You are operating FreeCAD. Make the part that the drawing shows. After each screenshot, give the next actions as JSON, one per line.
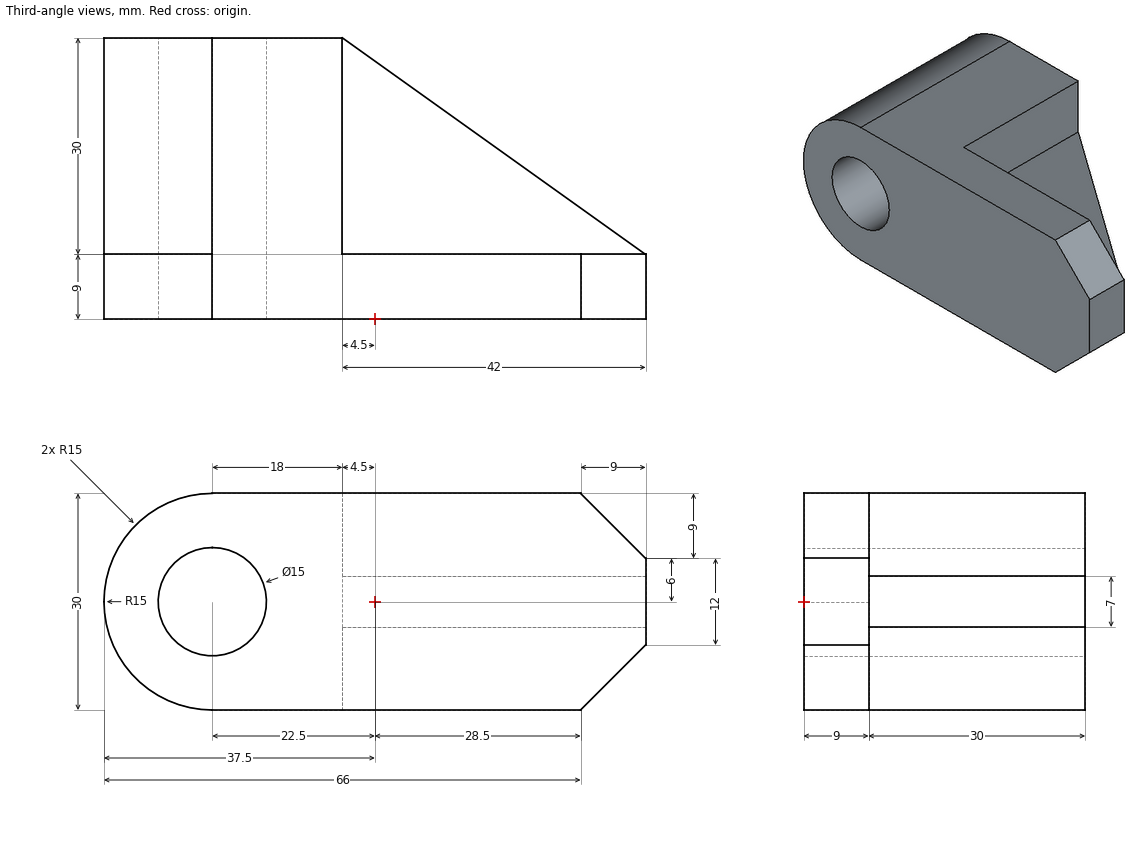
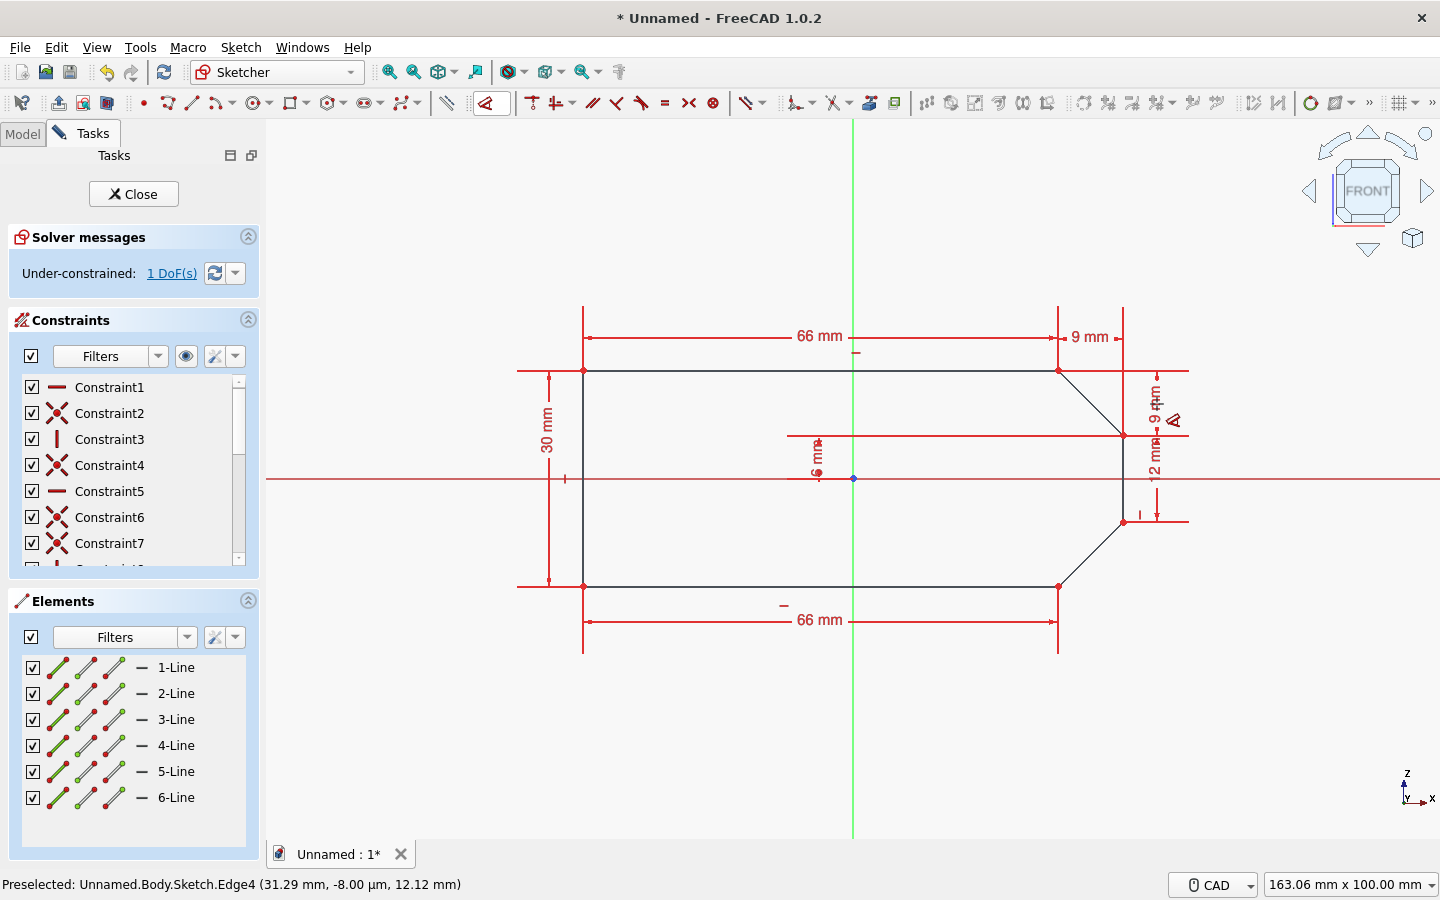
{"action": "left_click", "coordinate": [1058, 587]}
{"action": "left_click", "coordinate": [956, 621]}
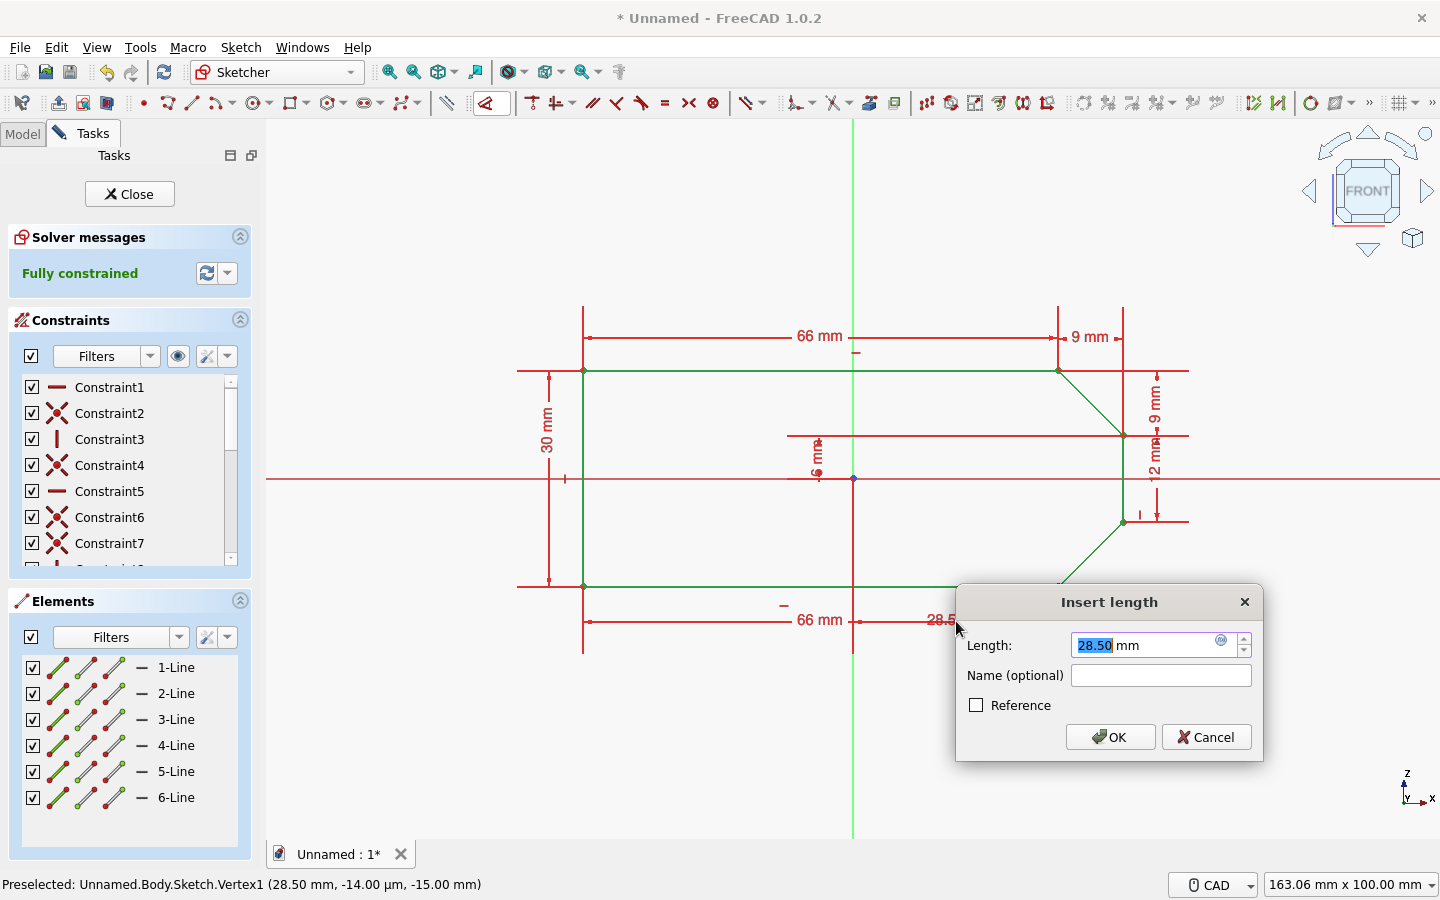
{"action": "type", "text": "28.5"}
{"action": "key", "text": "Return"}
{"action": "key", "text": "Escape"}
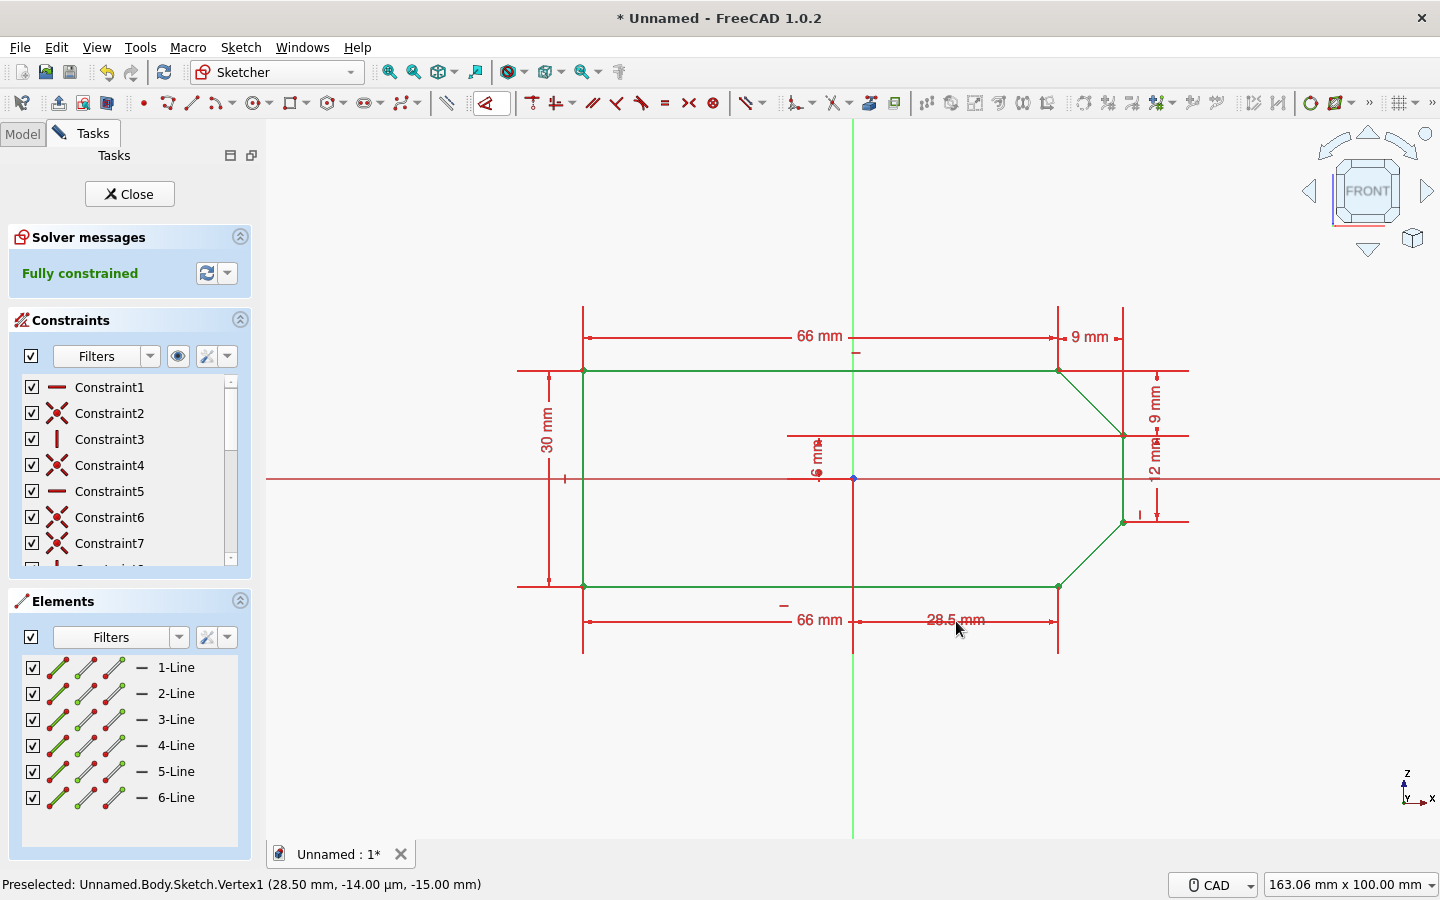
{"action": "left_click", "coordinate": [130, 194]}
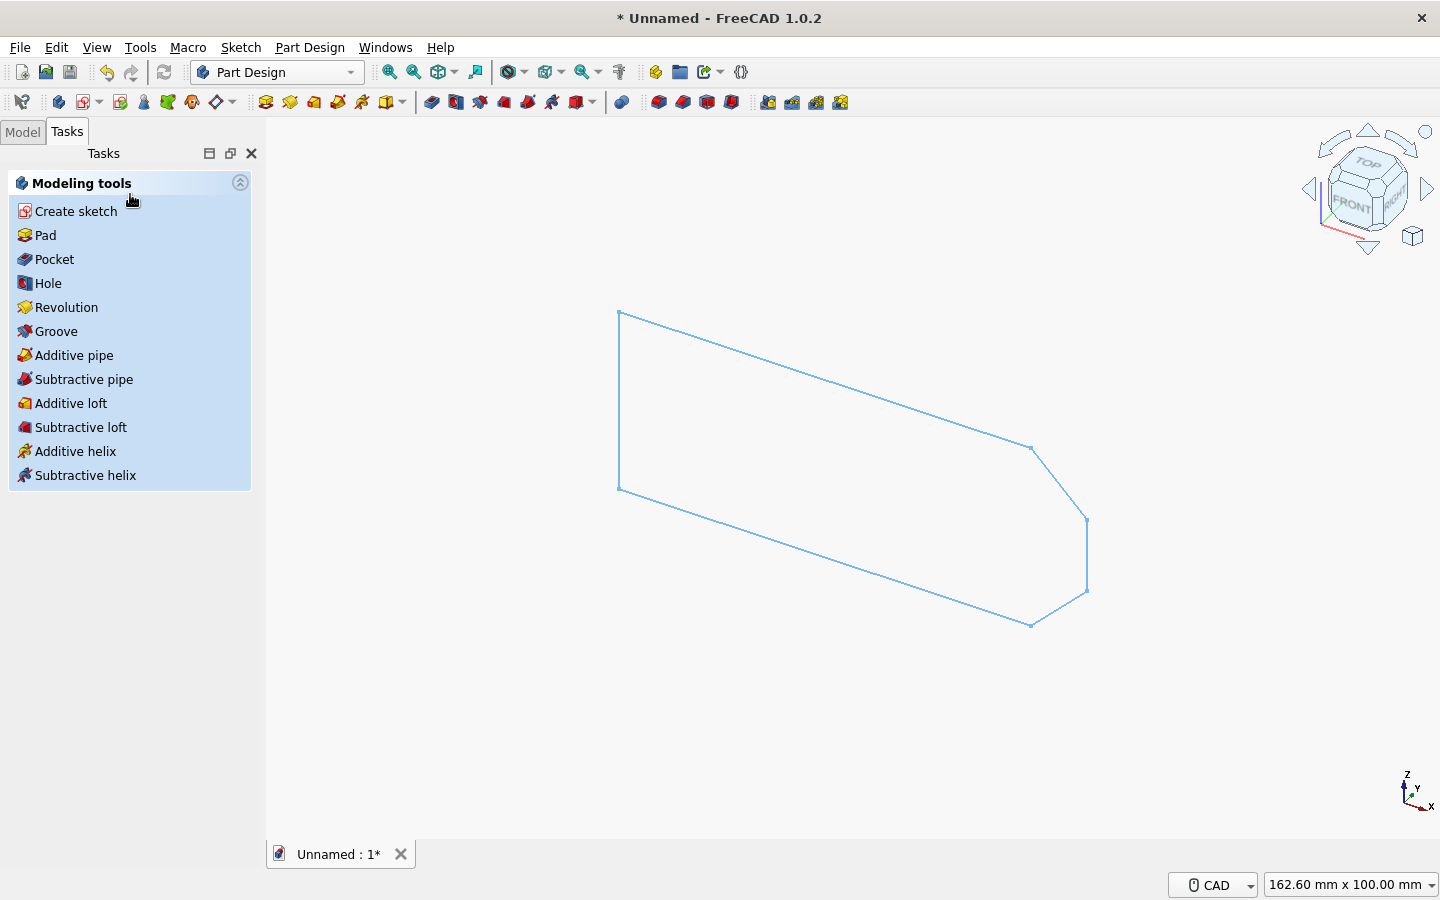
{"action": "left_click", "coordinate": [266, 102]}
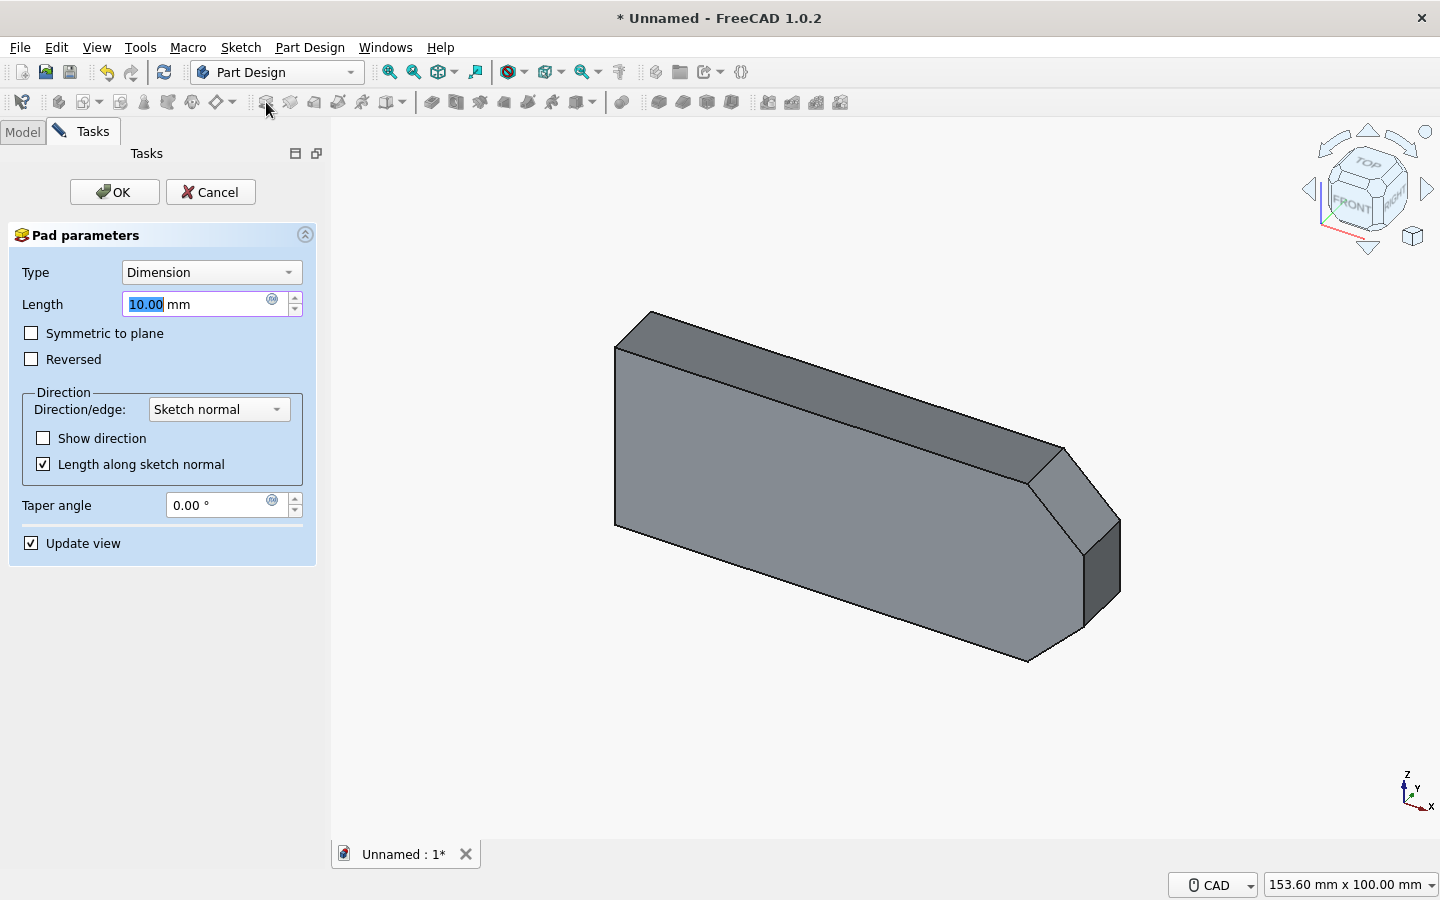
{"action": "type", "text": "9"}
{"action": "key", "text": "Tab"}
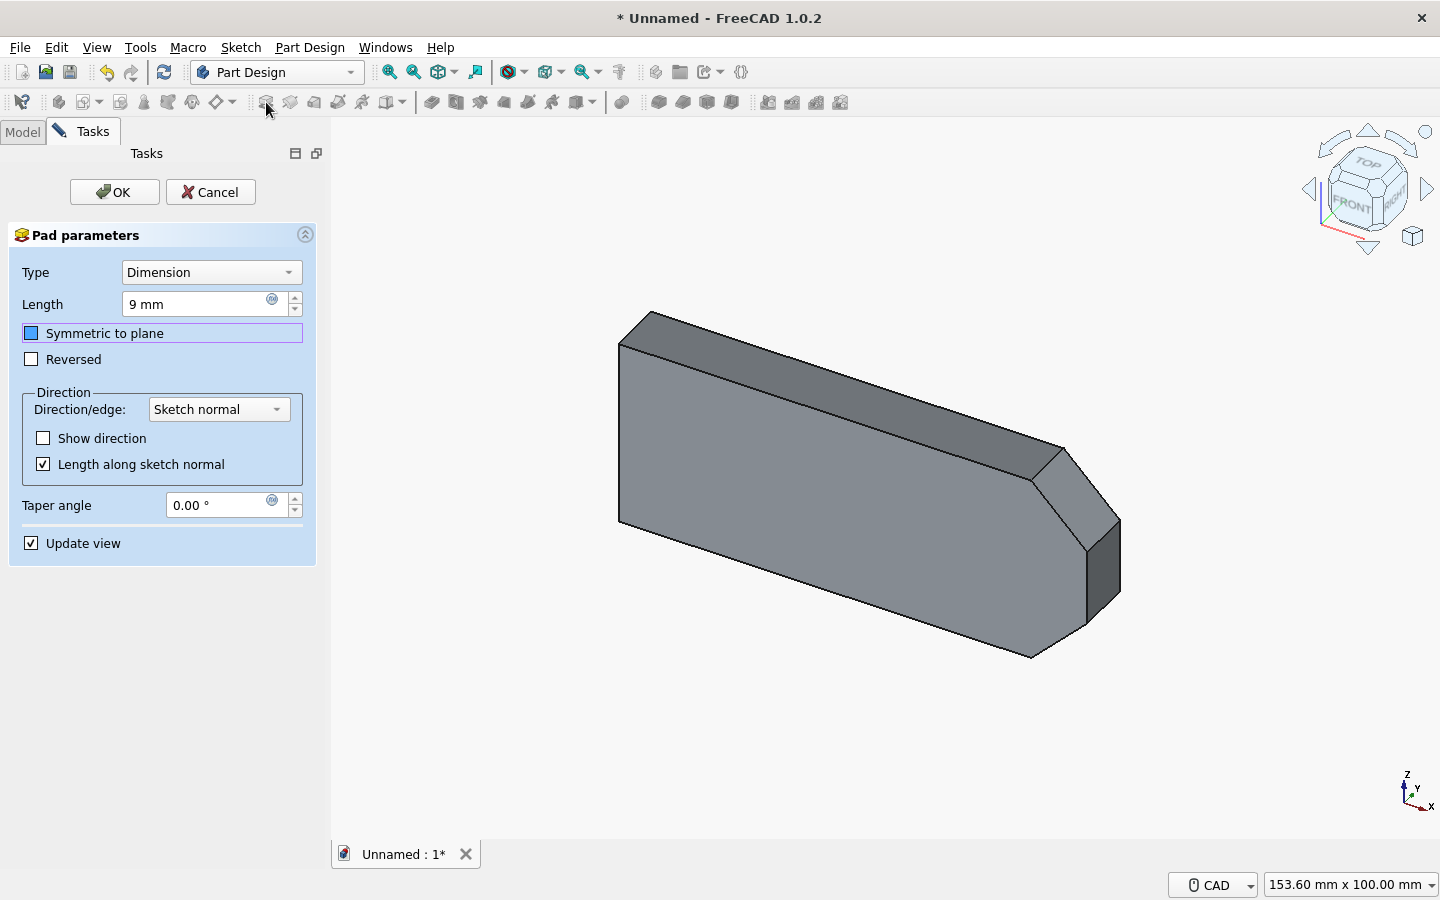
{"action": "left_click", "coordinate": [30, 359]}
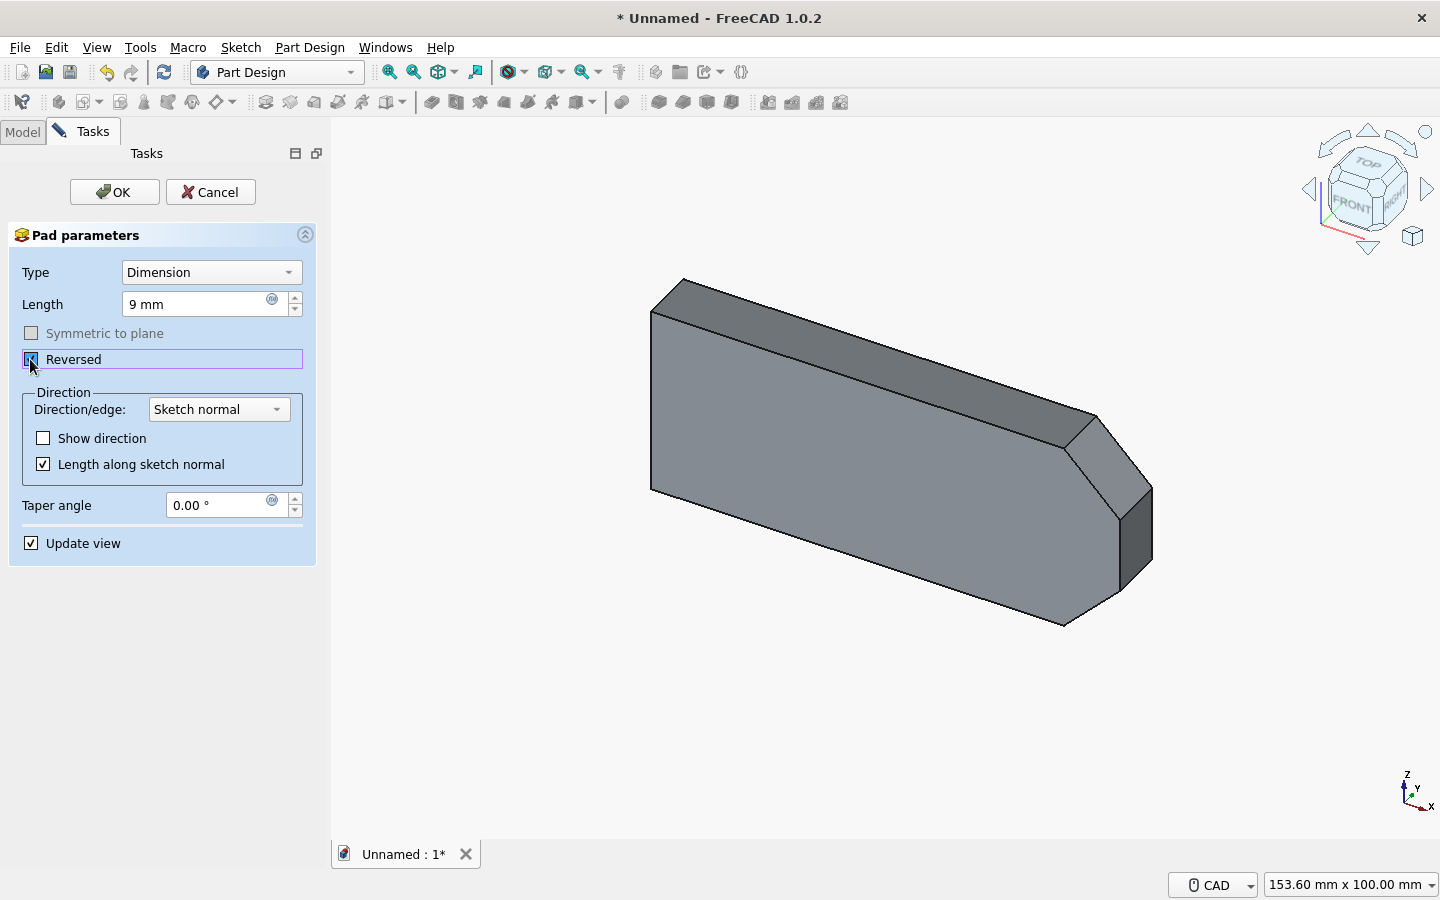
{"action": "left_click", "coordinate": [115, 192]}